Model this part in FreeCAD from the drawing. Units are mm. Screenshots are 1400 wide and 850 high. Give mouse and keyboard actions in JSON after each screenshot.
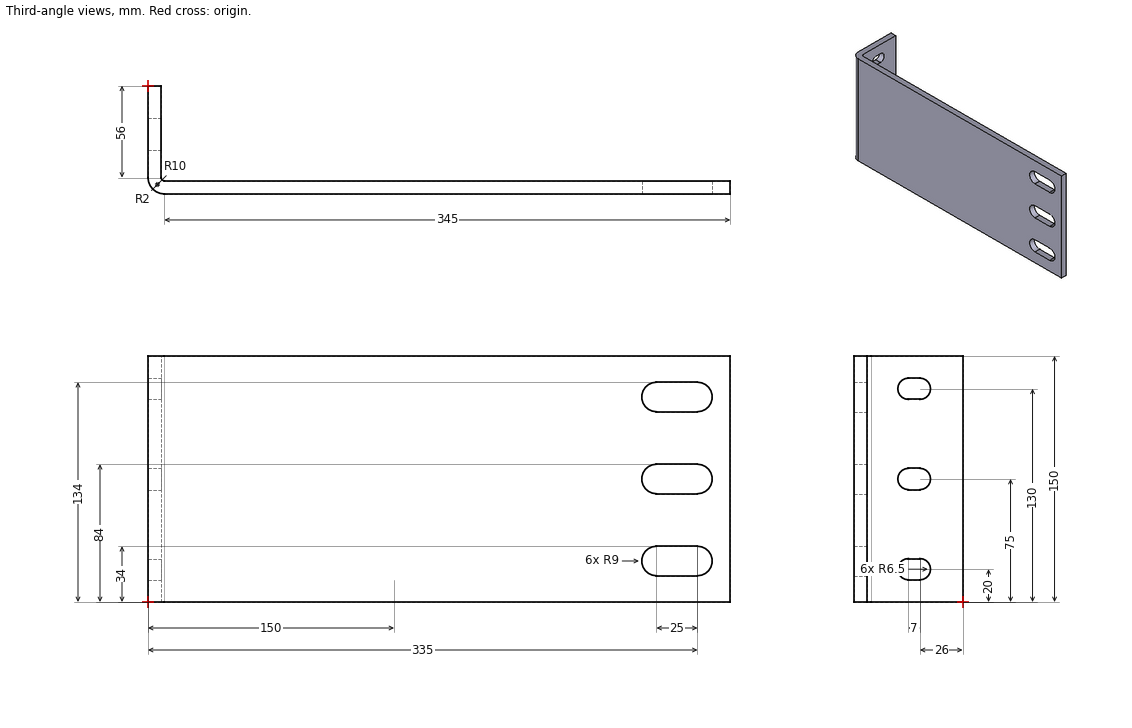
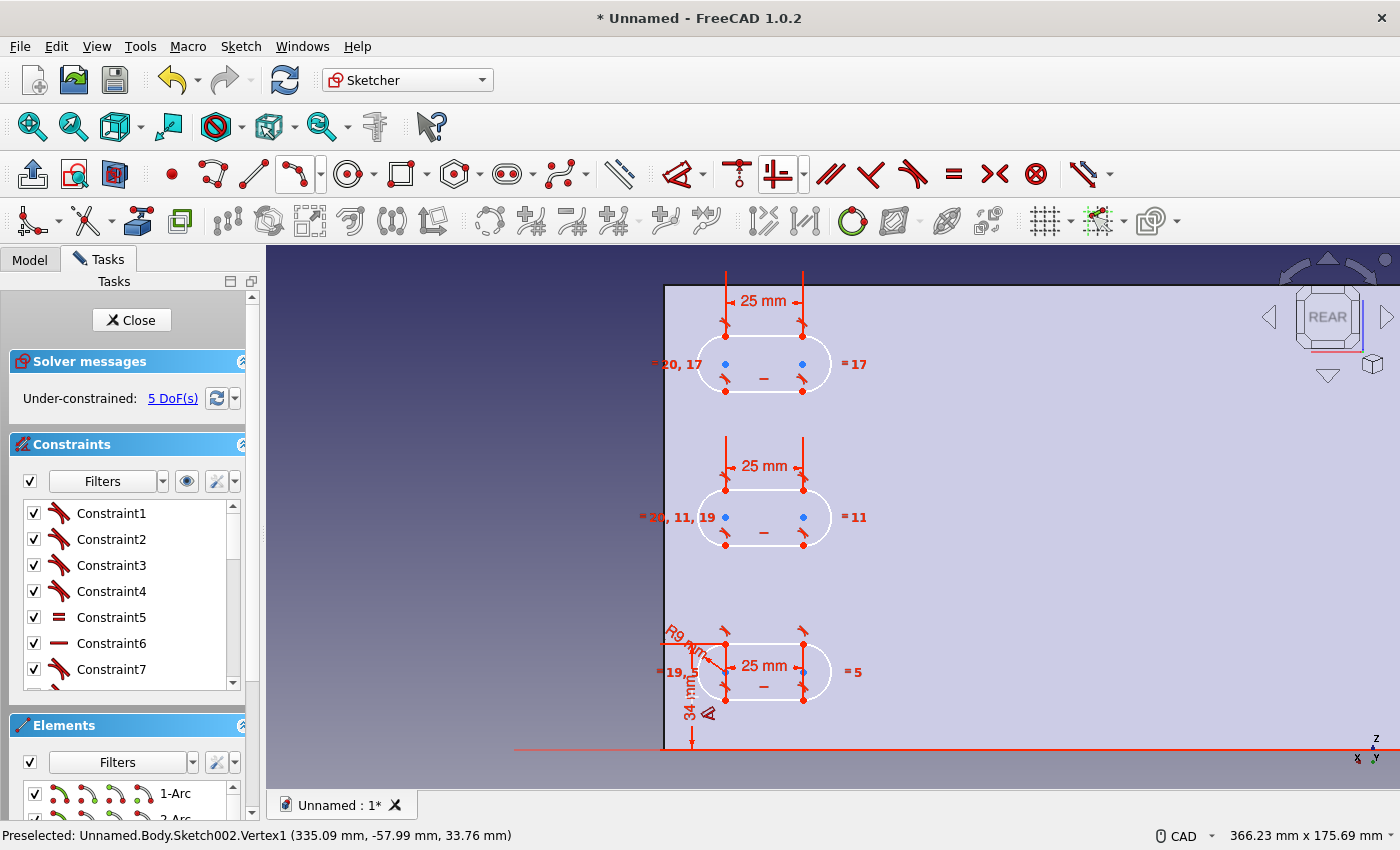
{"action": "left_click", "coordinate": [726, 490]}
{"action": "left_click", "coordinate": [692, 620]}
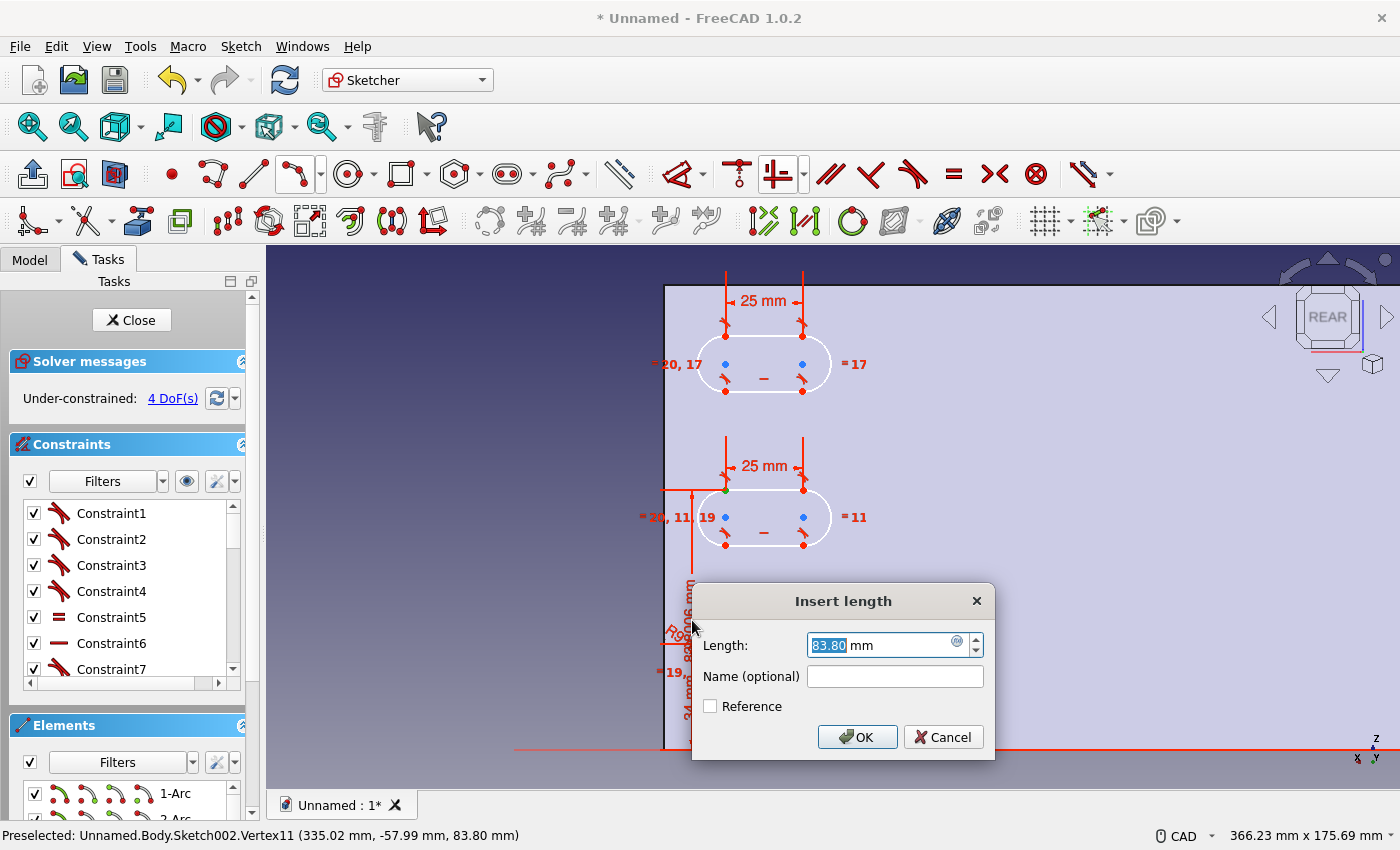
{"action": "type", "text": "84"}
{"action": "key", "text": "Return"}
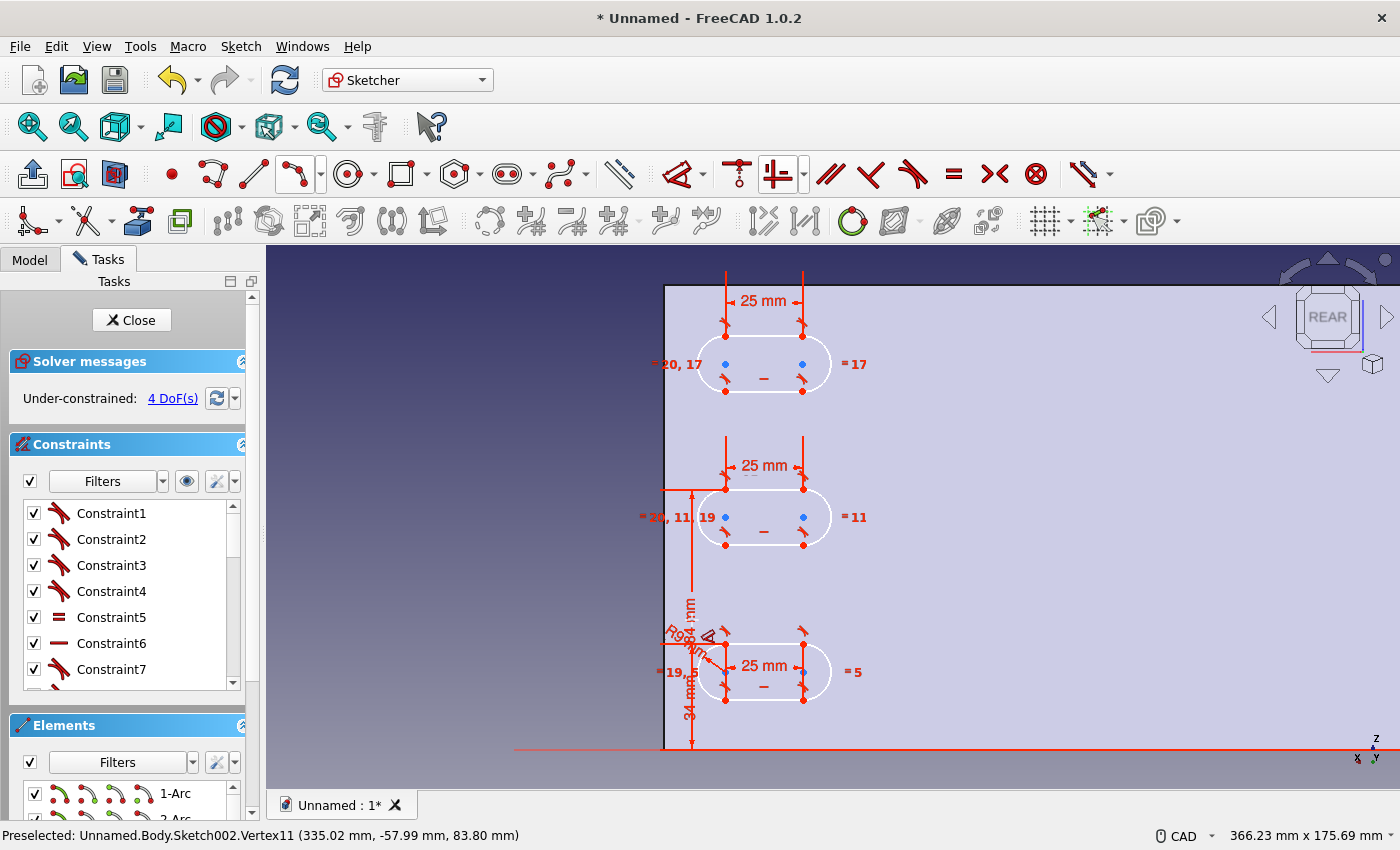
{"action": "left_click", "coordinate": [726, 644]}
{"action": "left_click", "coordinate": [980, 610]}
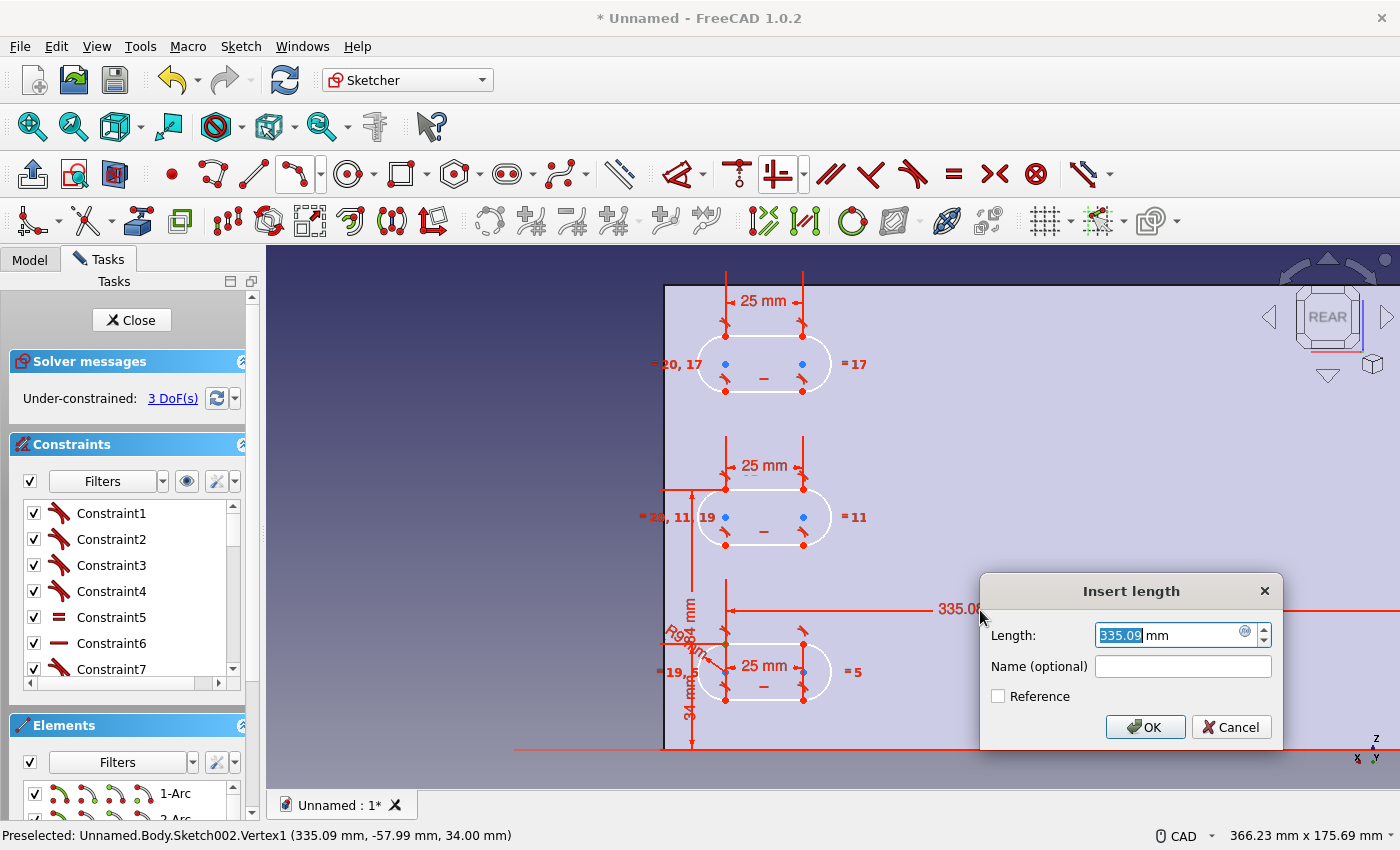
{"action": "type", "text": "335"}
{"action": "key", "text": "Return"}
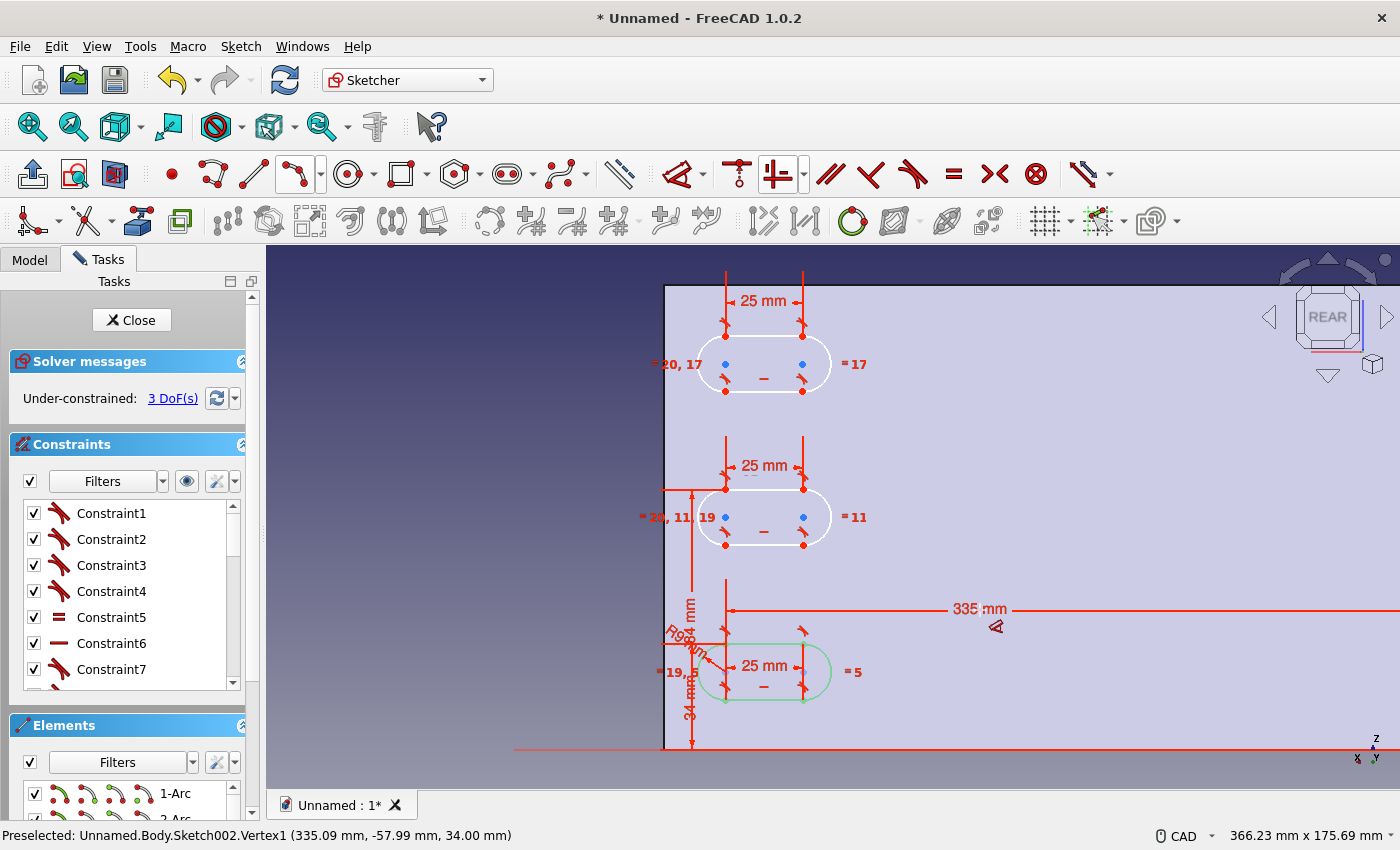
{"action": "left_click", "coordinate": [726, 490]}
{"action": "left_click", "coordinate": [980, 456]}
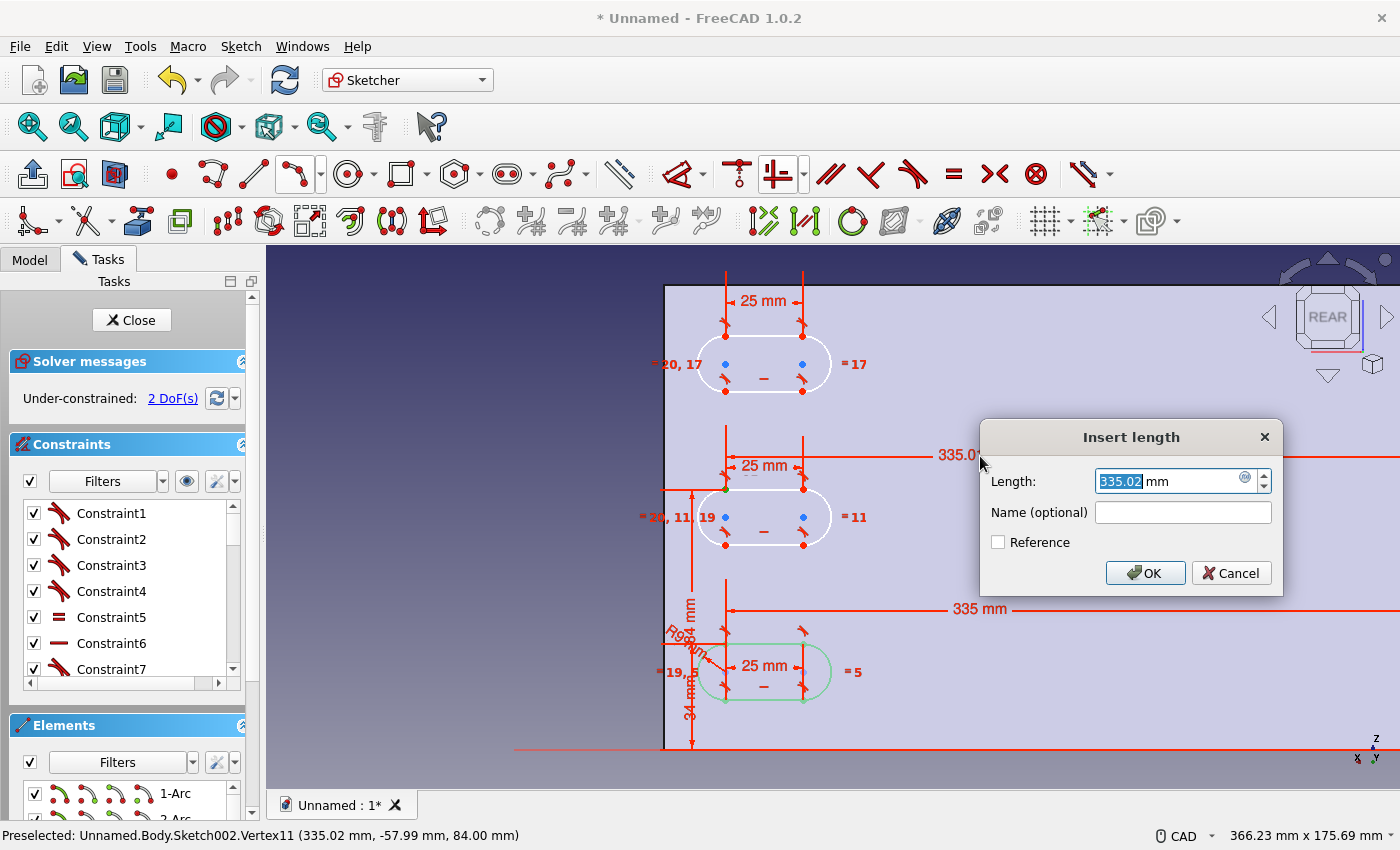
{"action": "type", "text": "335"}
{"action": "key", "text": "Return"}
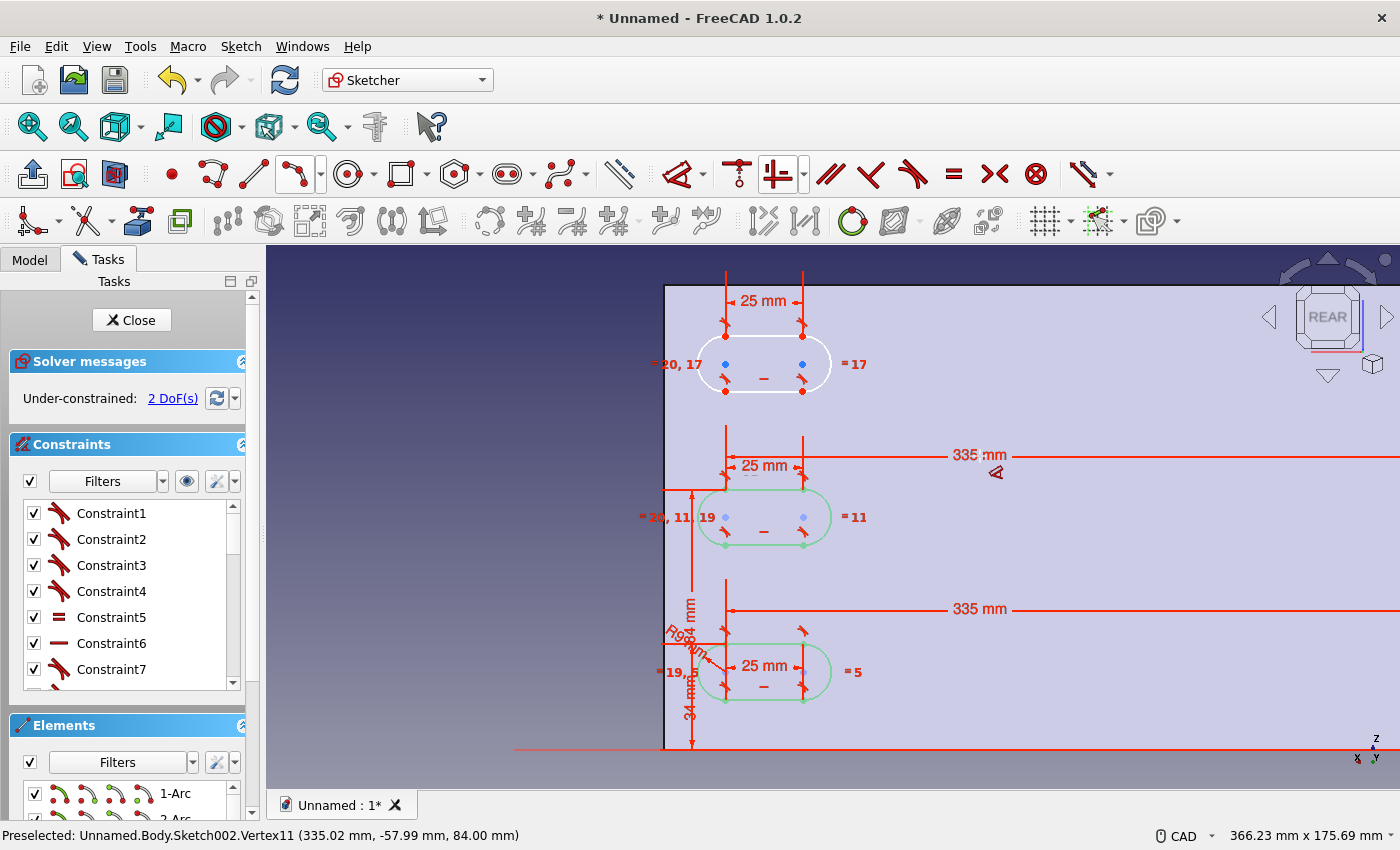
{"action": "left_click", "coordinate": [726, 336]}
{"action": "left_click", "coordinate": [980, 302]}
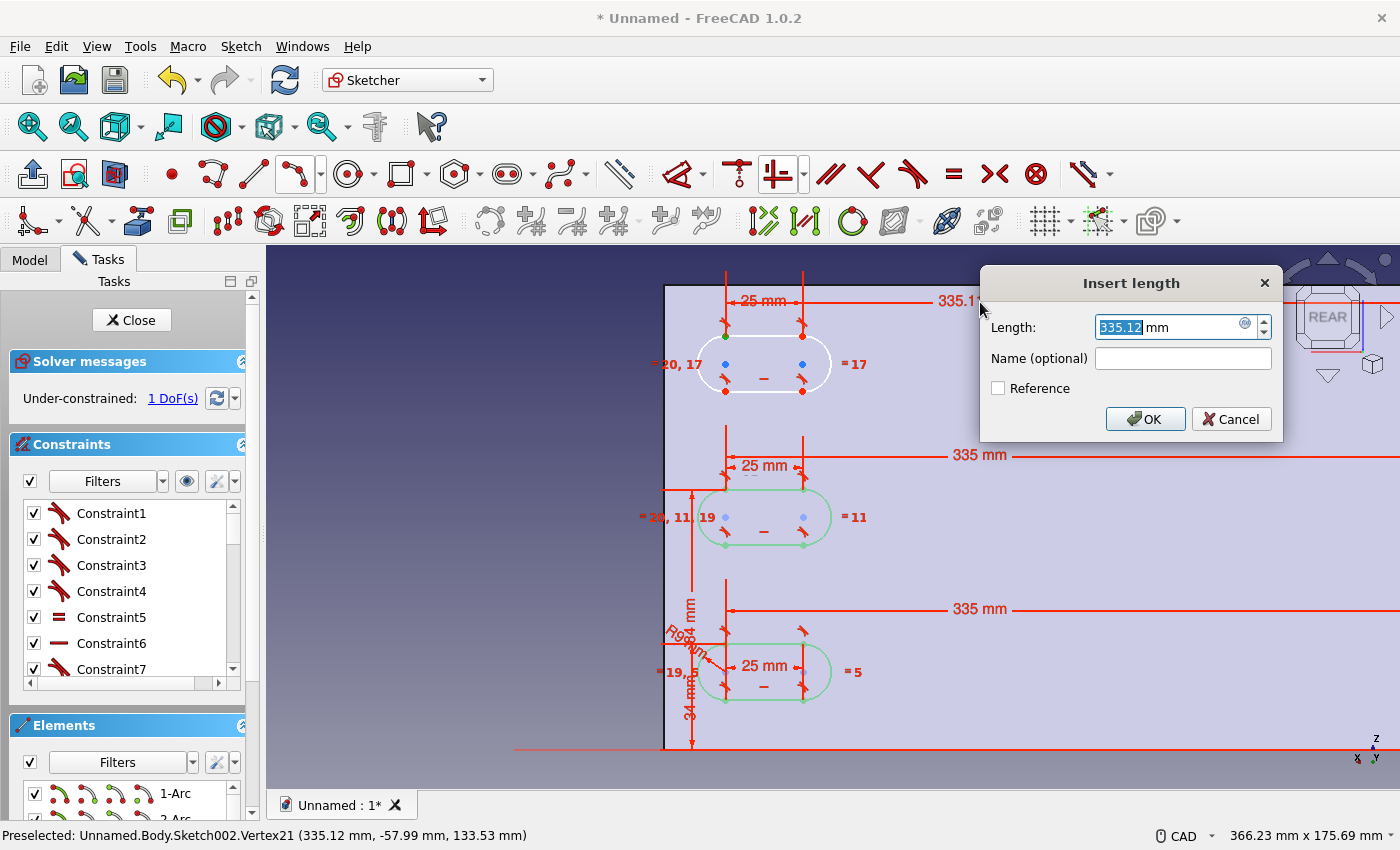
{"action": "type", "text": "335"}
{"action": "key", "text": "Return"}